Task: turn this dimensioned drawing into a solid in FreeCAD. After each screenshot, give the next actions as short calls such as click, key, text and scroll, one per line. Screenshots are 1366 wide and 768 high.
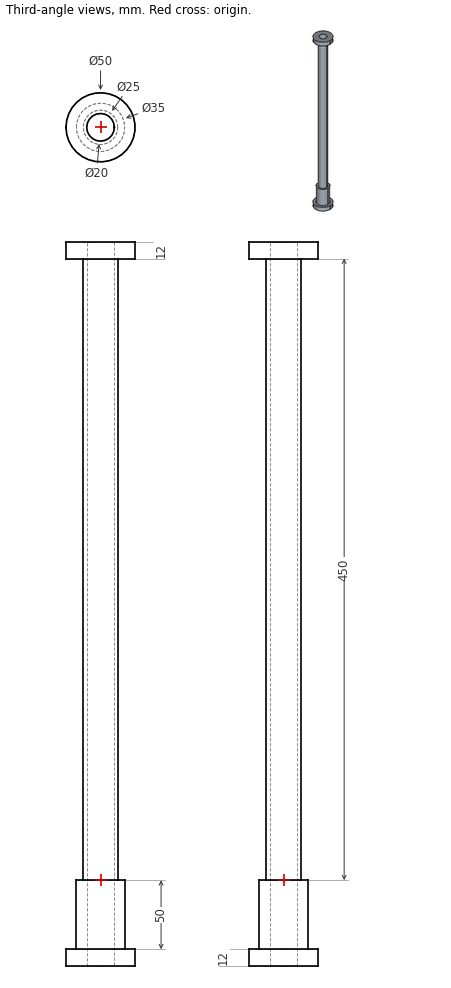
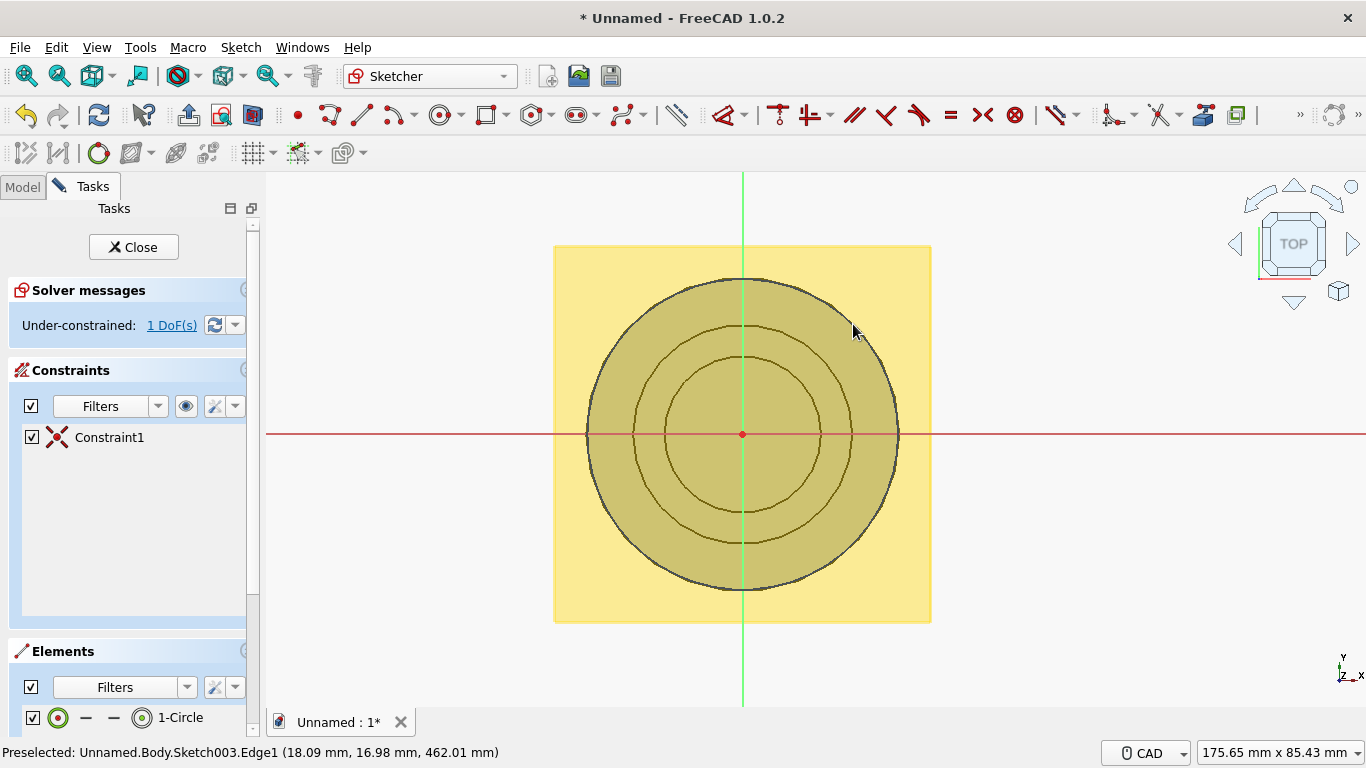
click(724, 116)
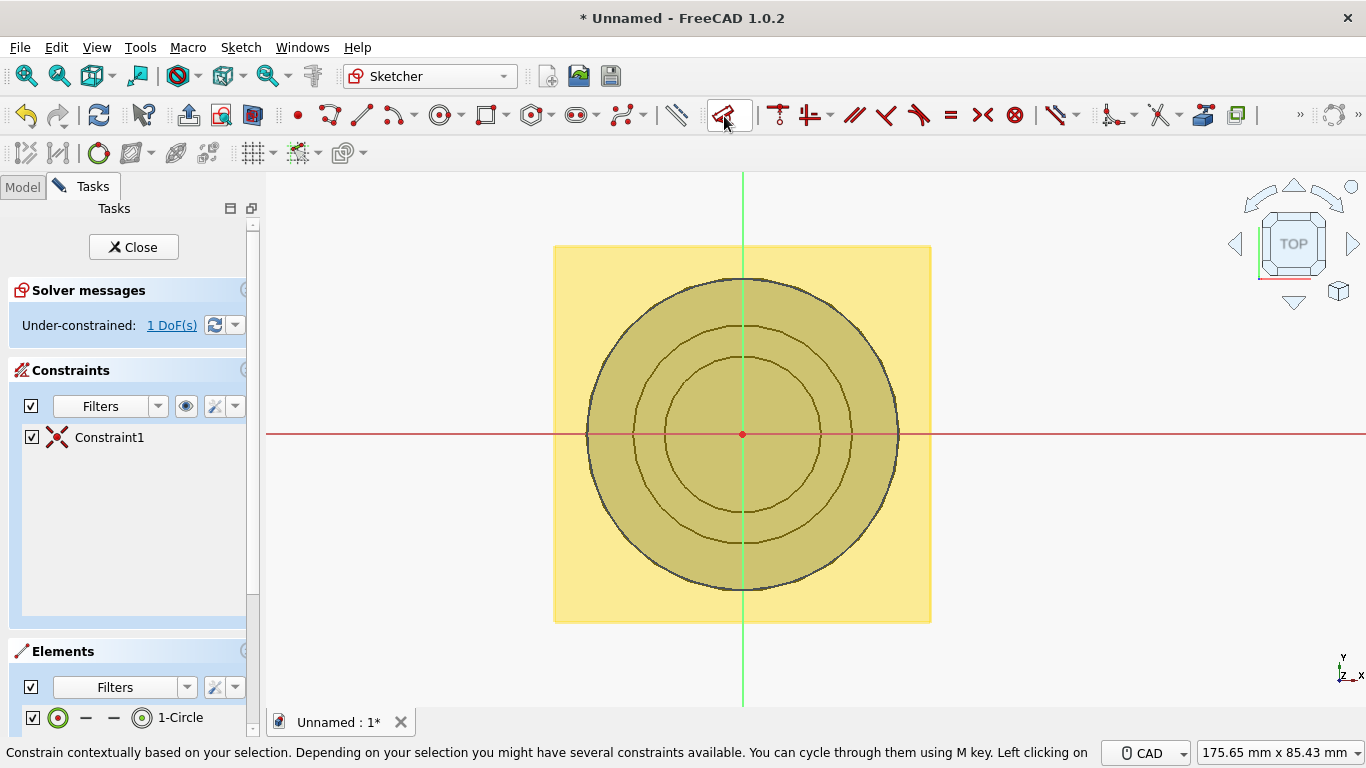
click(852, 324)
click(875, 301)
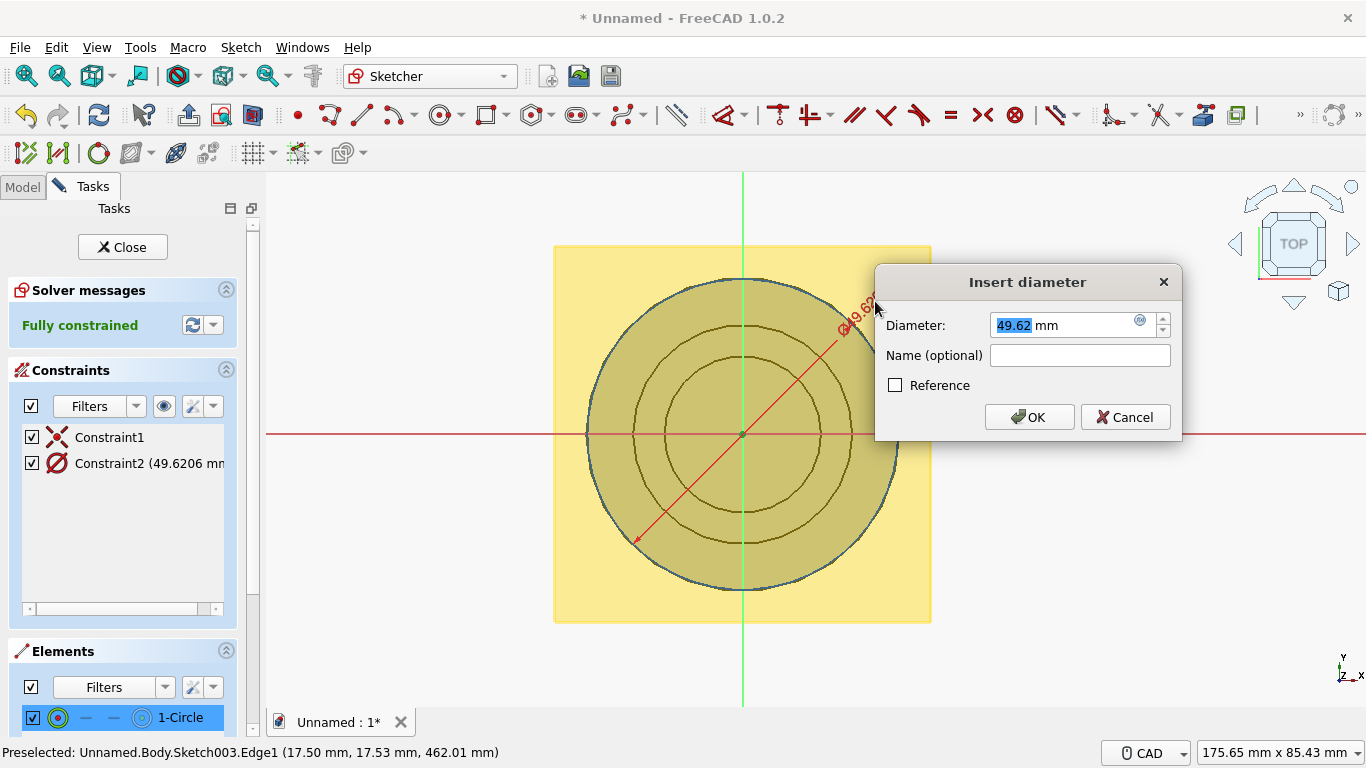
text(50)
key(Return)
key(Escape)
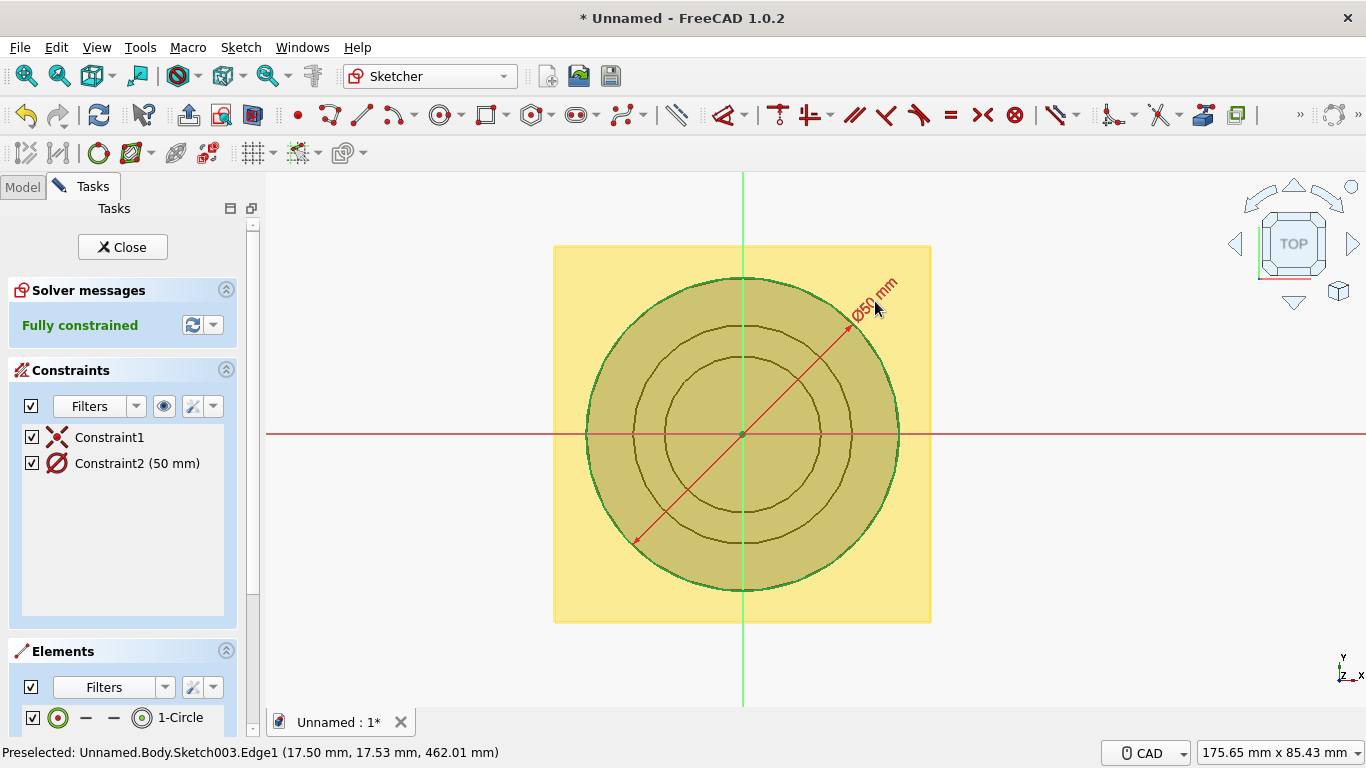
click(123, 247)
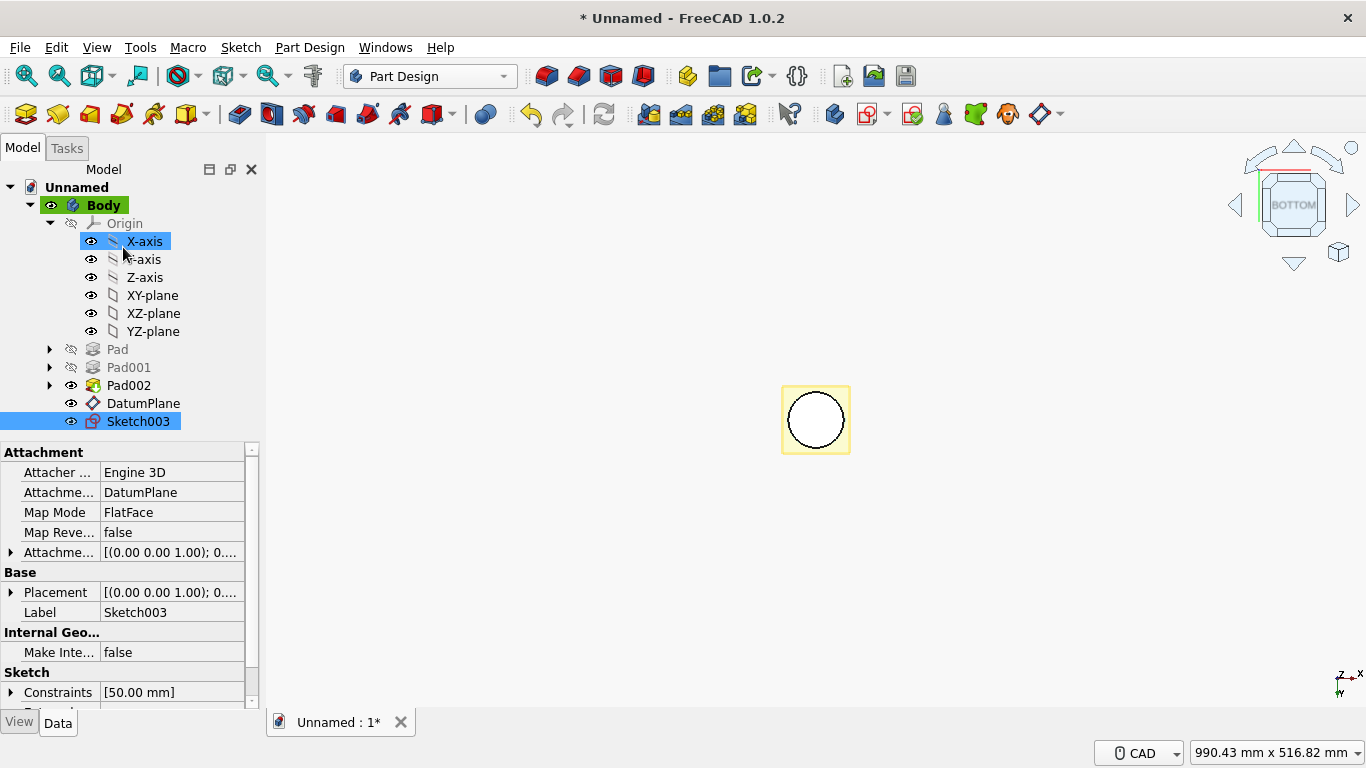
click(26, 114)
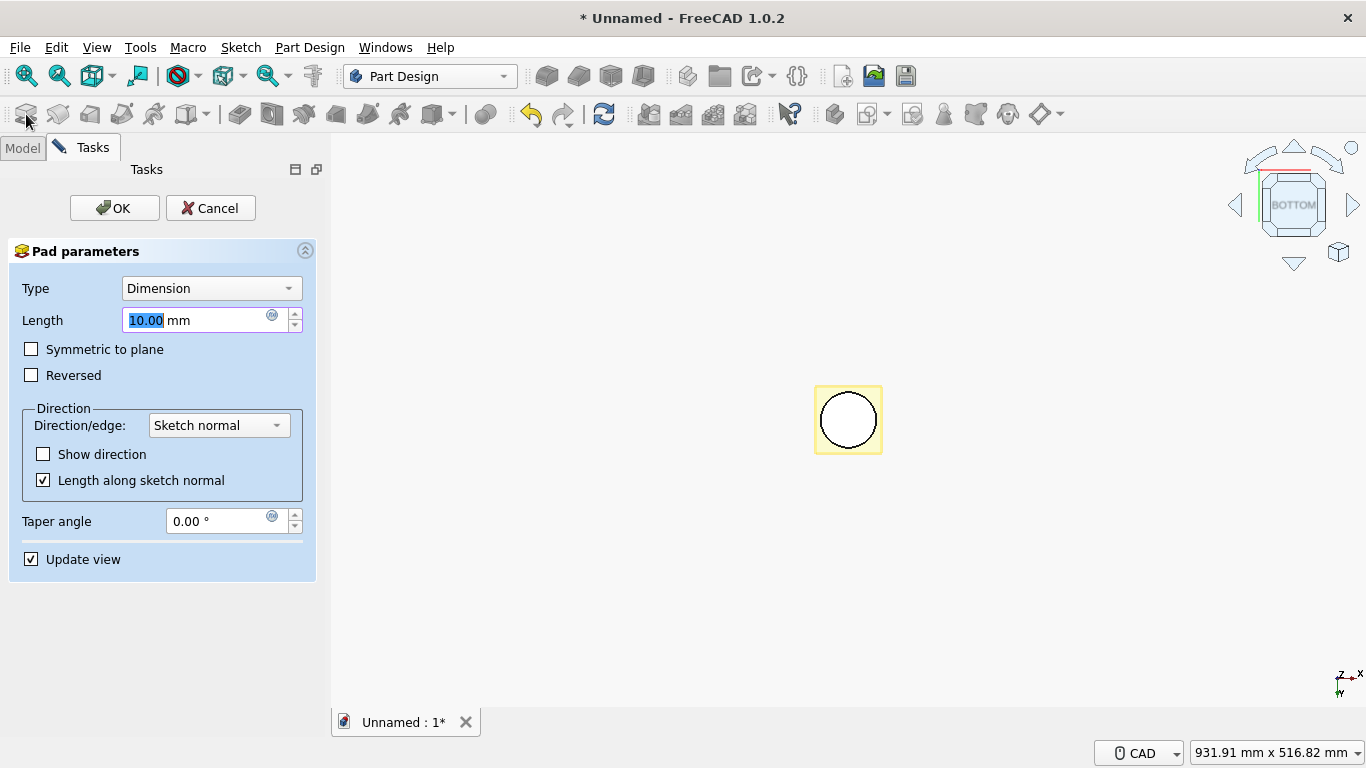
text(12)
key(Tab)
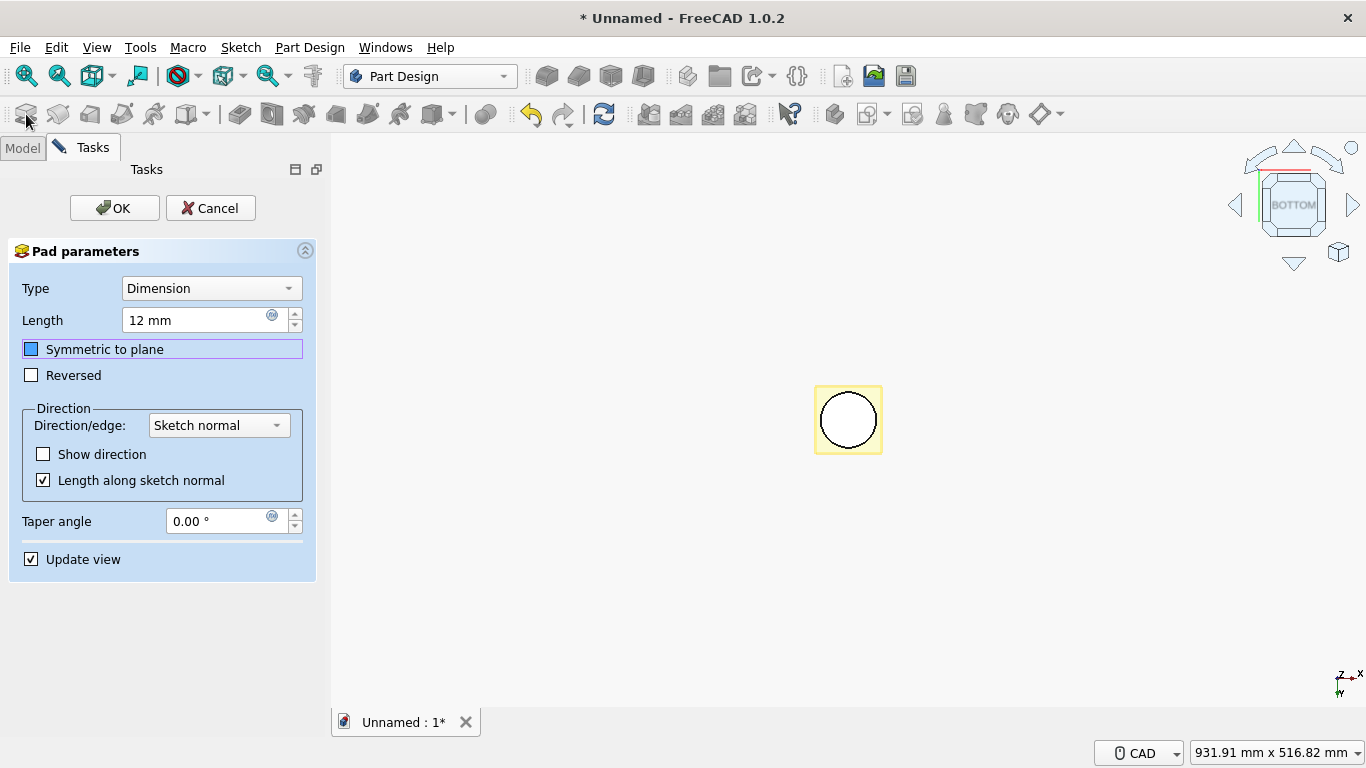
click(30, 375)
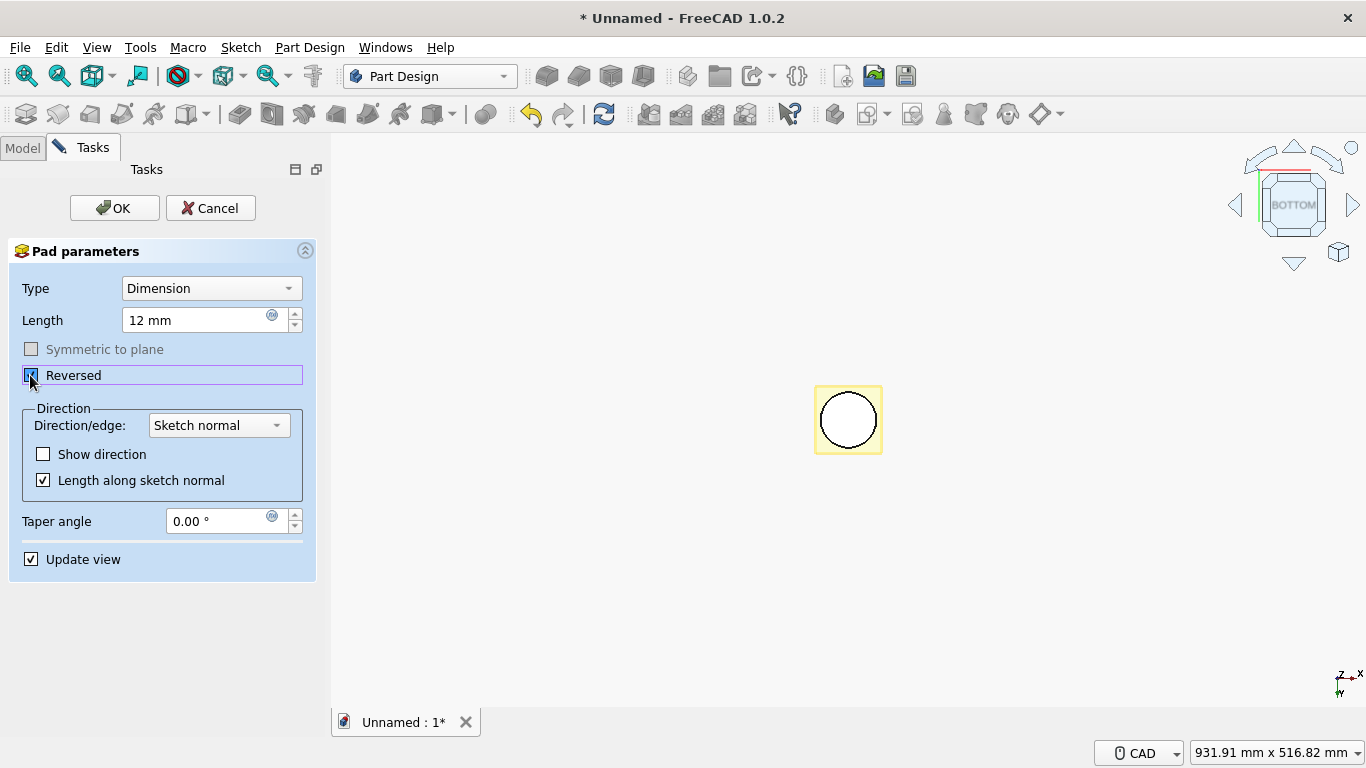
click(115, 208)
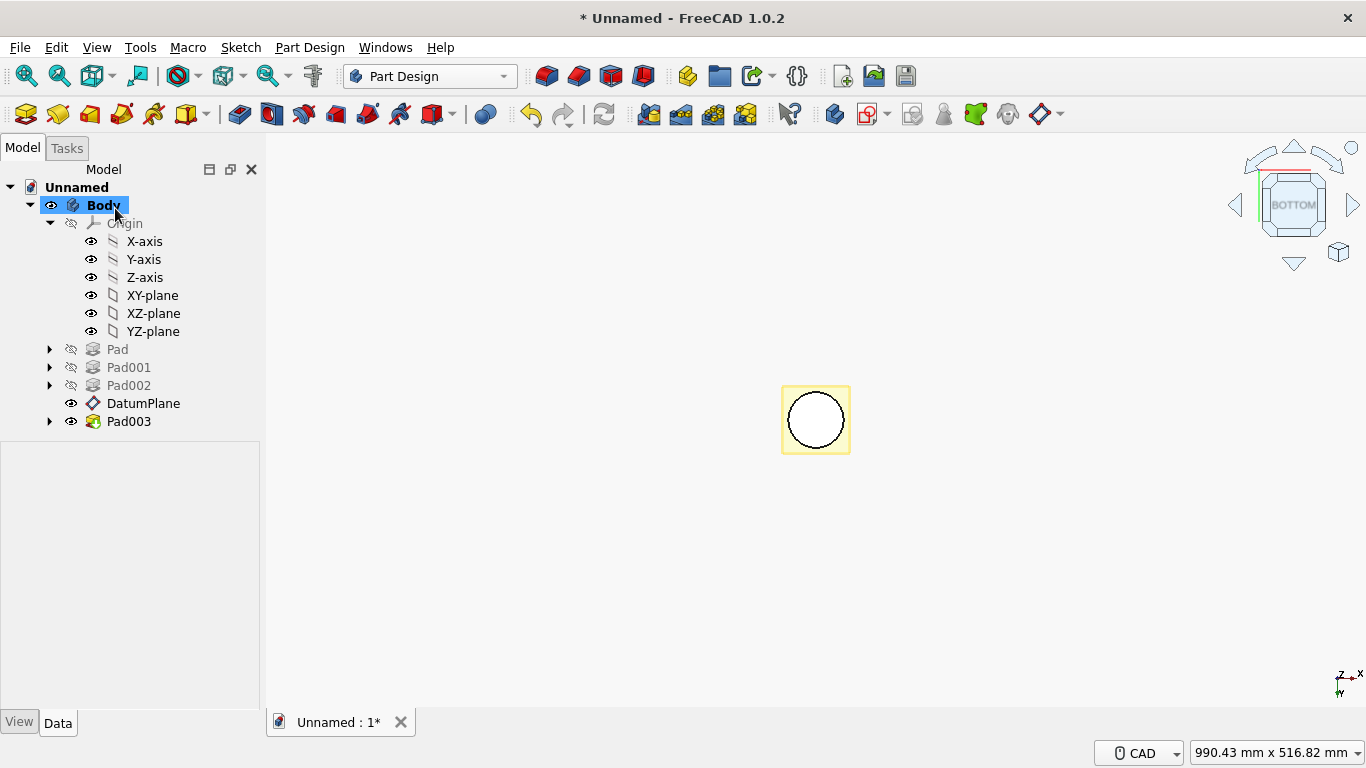
click(116, 403)
key(space)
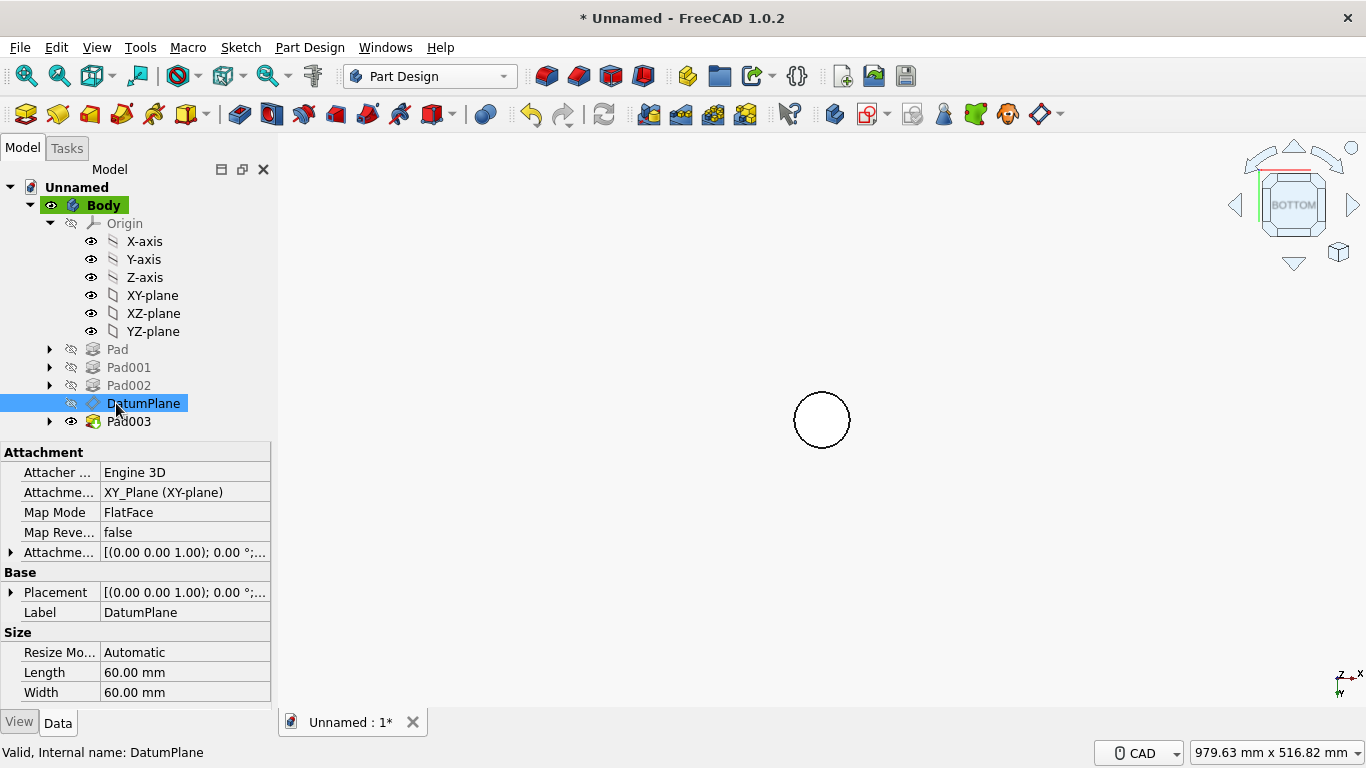
key(v)
key(f)